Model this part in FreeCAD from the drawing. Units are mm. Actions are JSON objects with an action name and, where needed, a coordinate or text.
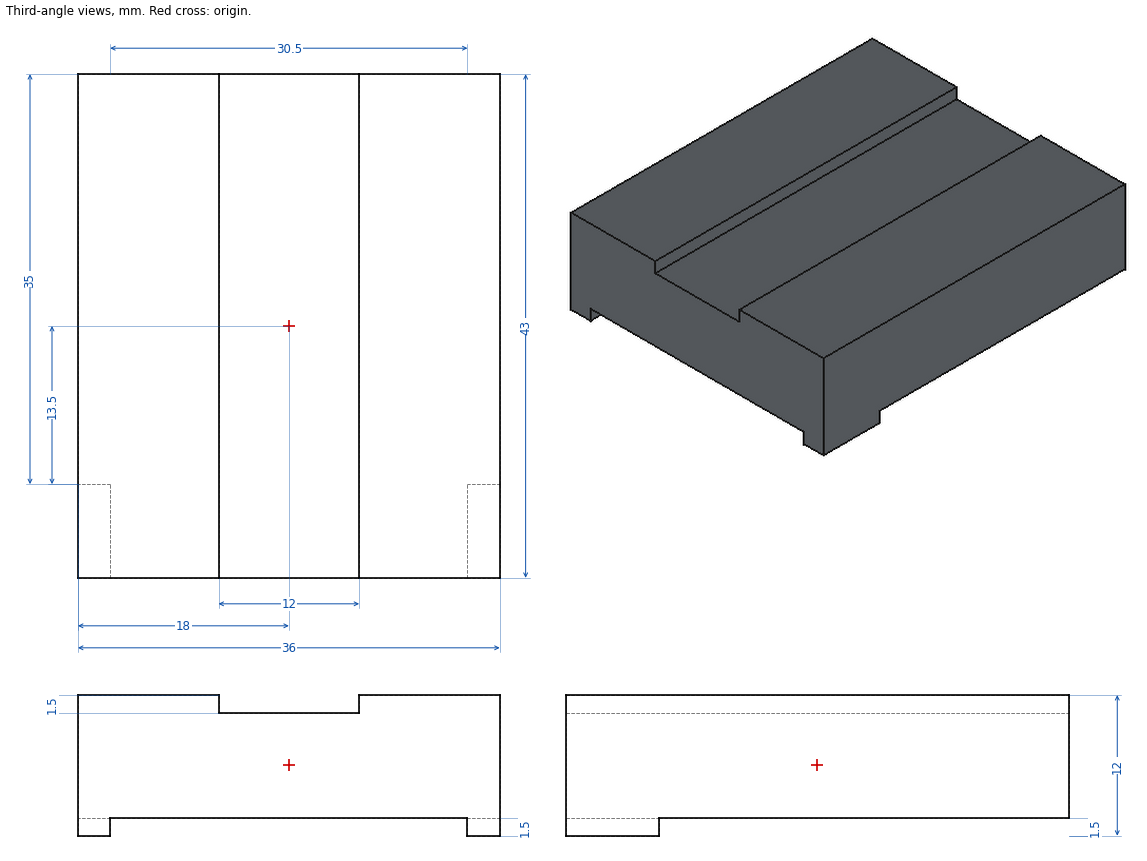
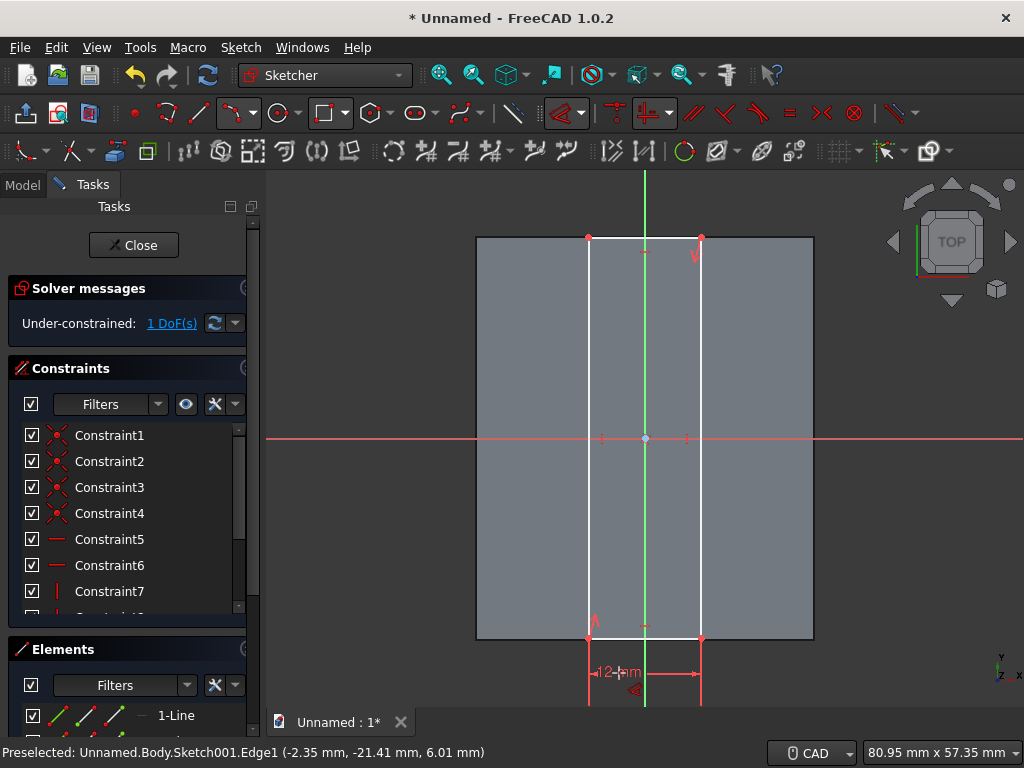
{"action": "left_click", "coordinate": [701, 519]}
{"action": "left_click", "coordinate": [735, 346]}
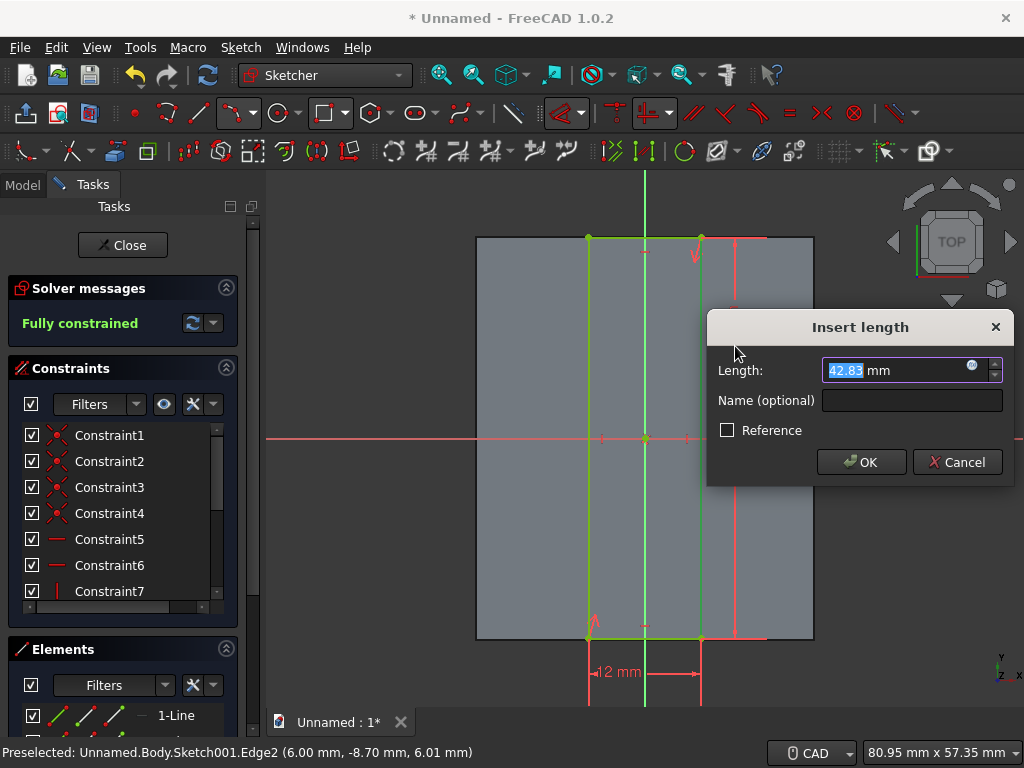
{"action": "type", "text": "43"}
{"action": "key", "text": "Return"}
{"action": "key", "text": "Escape"}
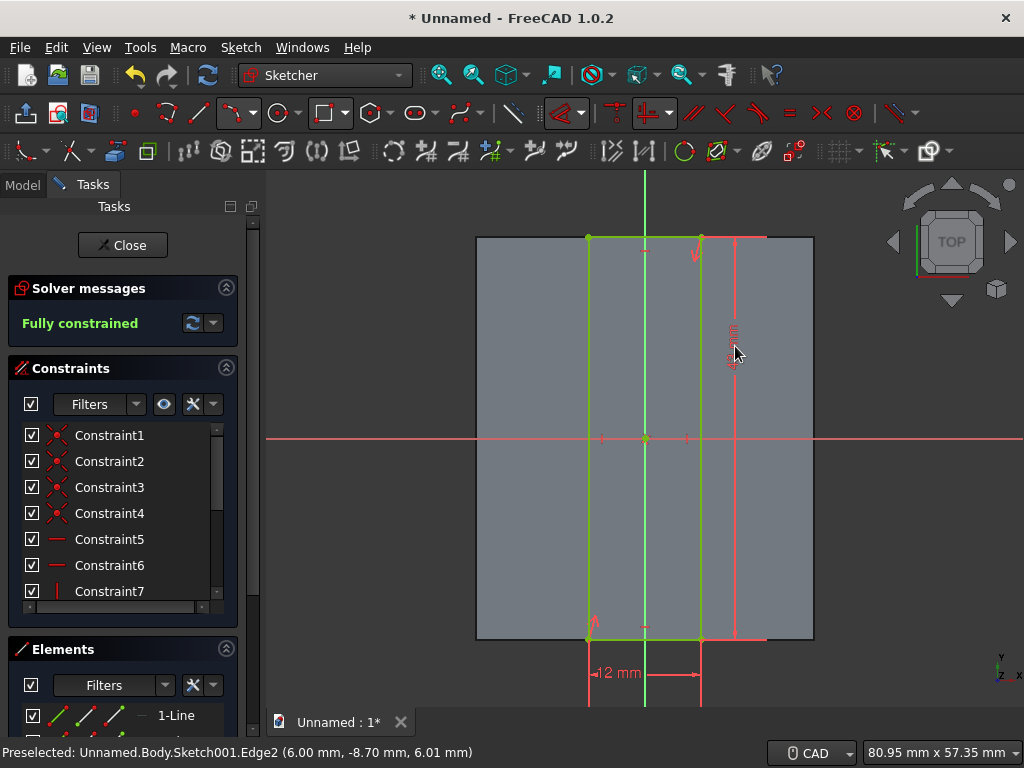
{"action": "left_click", "coordinate": [123, 245]}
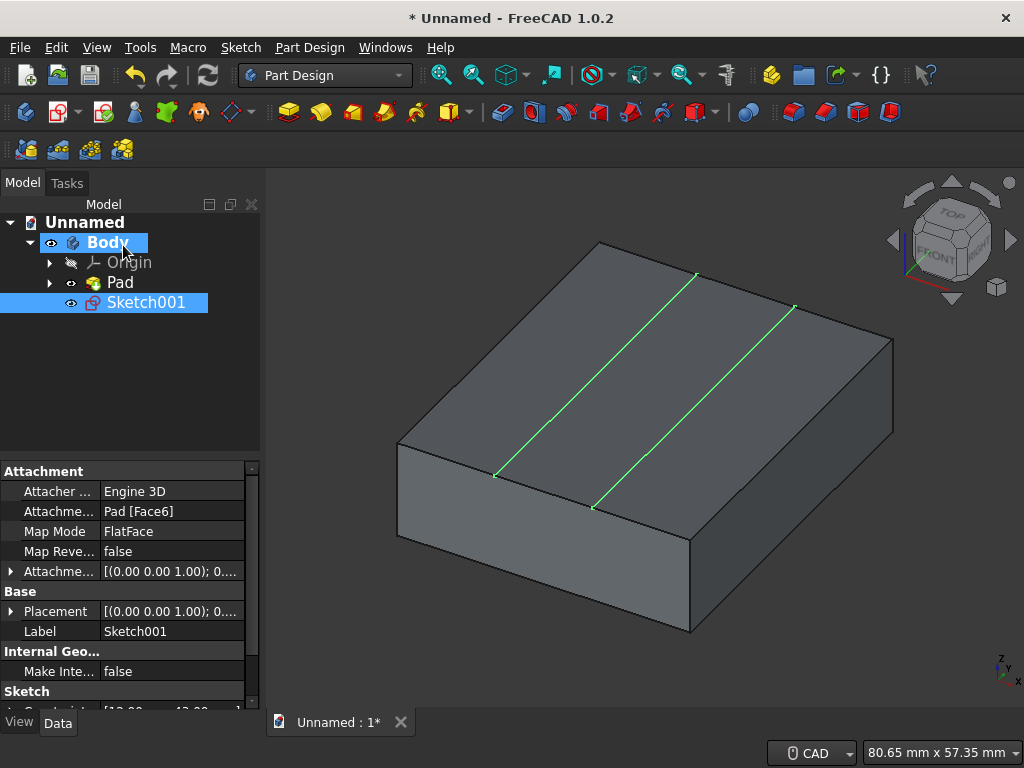
{"action": "left_click", "coordinate": [504, 112]}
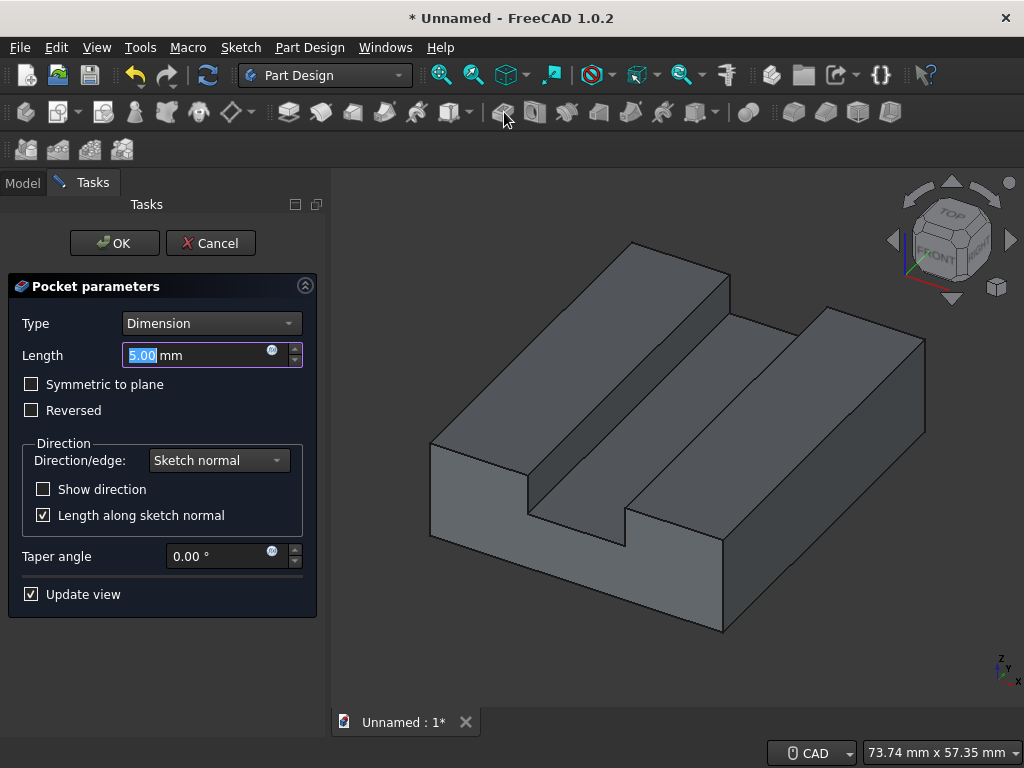
{"action": "type", "text": "1.5"}
{"action": "key", "text": "Tab"}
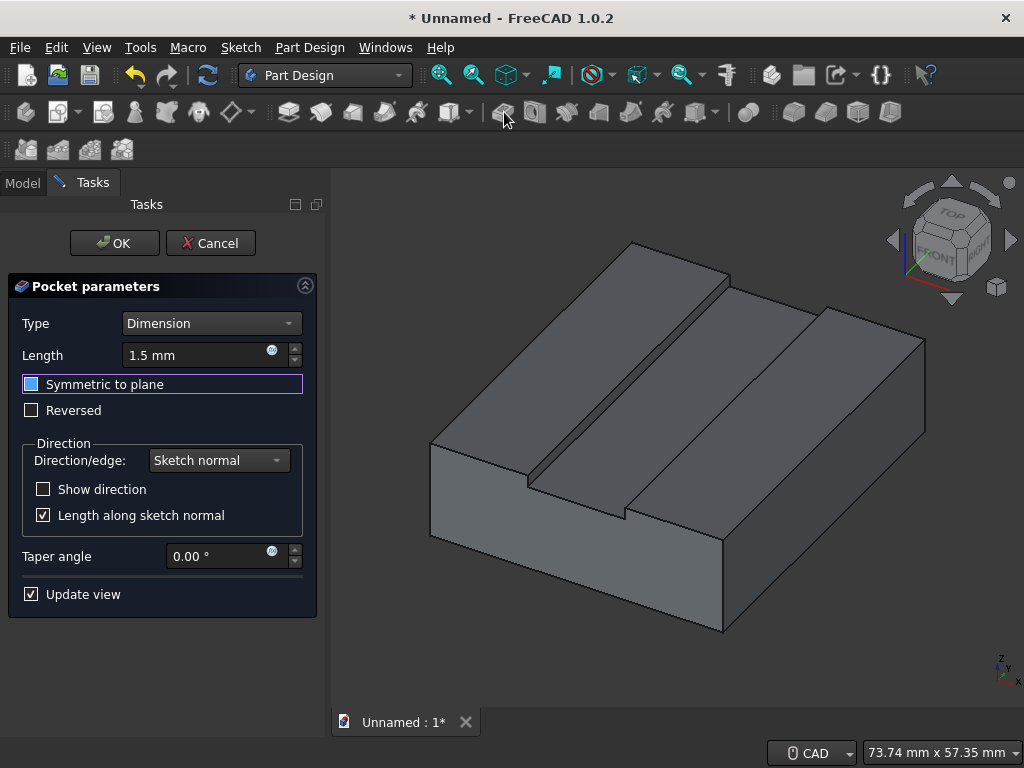
{"action": "left_click", "coordinate": [115, 243]}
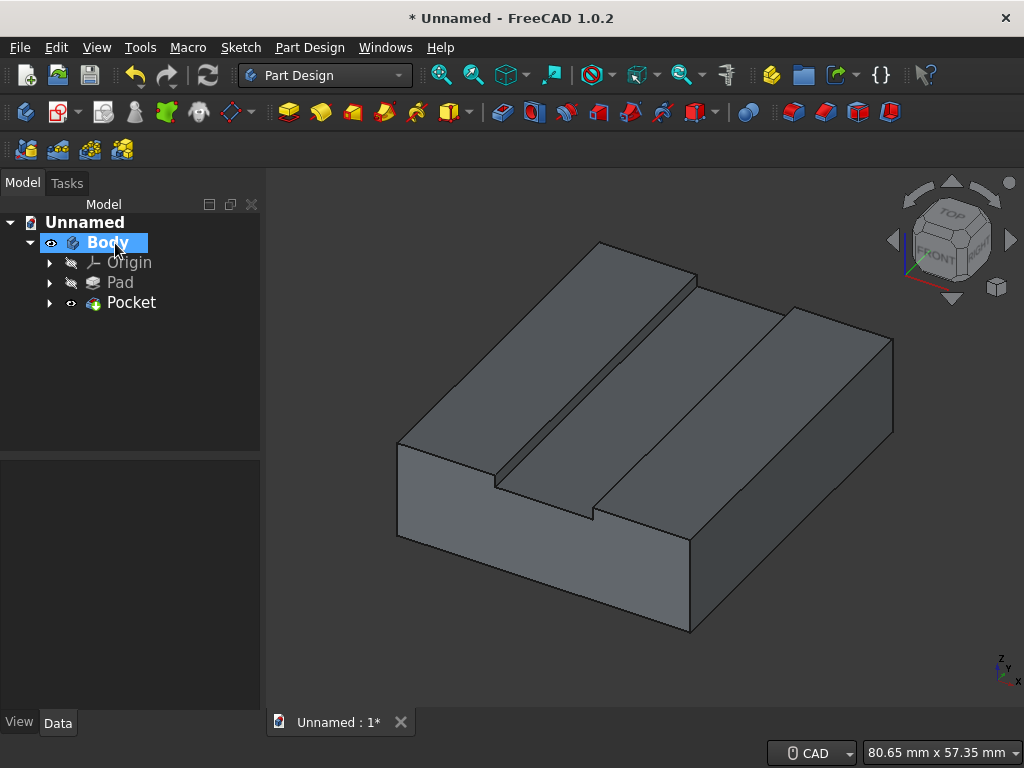
{"action": "key", "text": "5"}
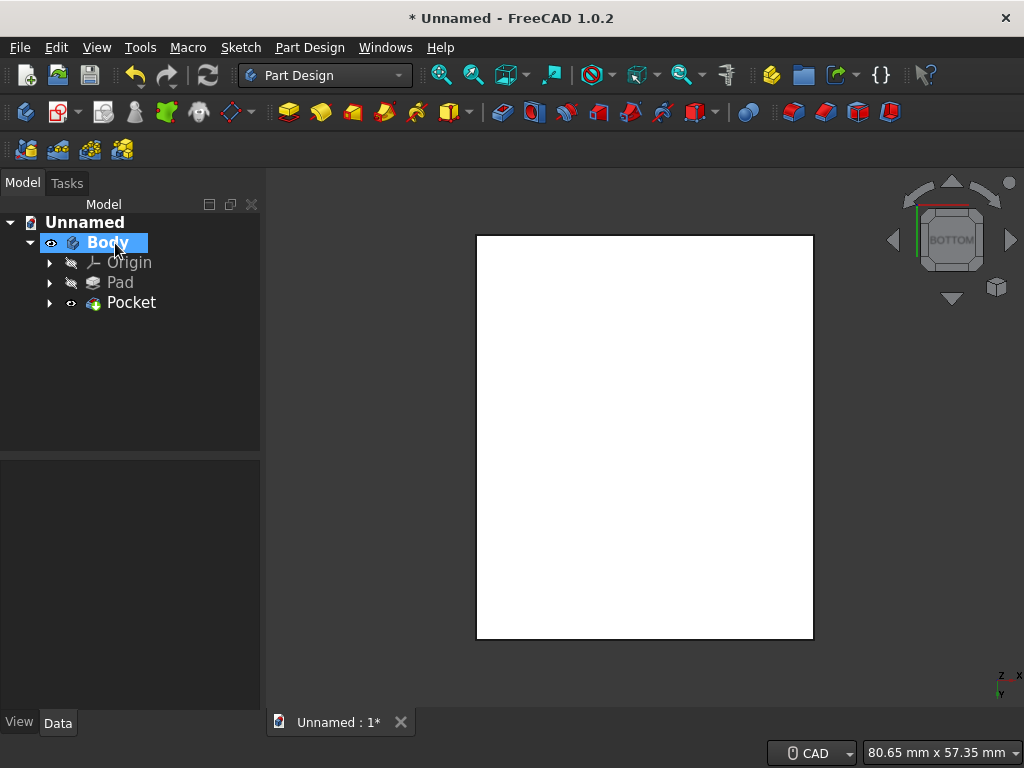
{"action": "left_click", "coordinate": [645, 436]}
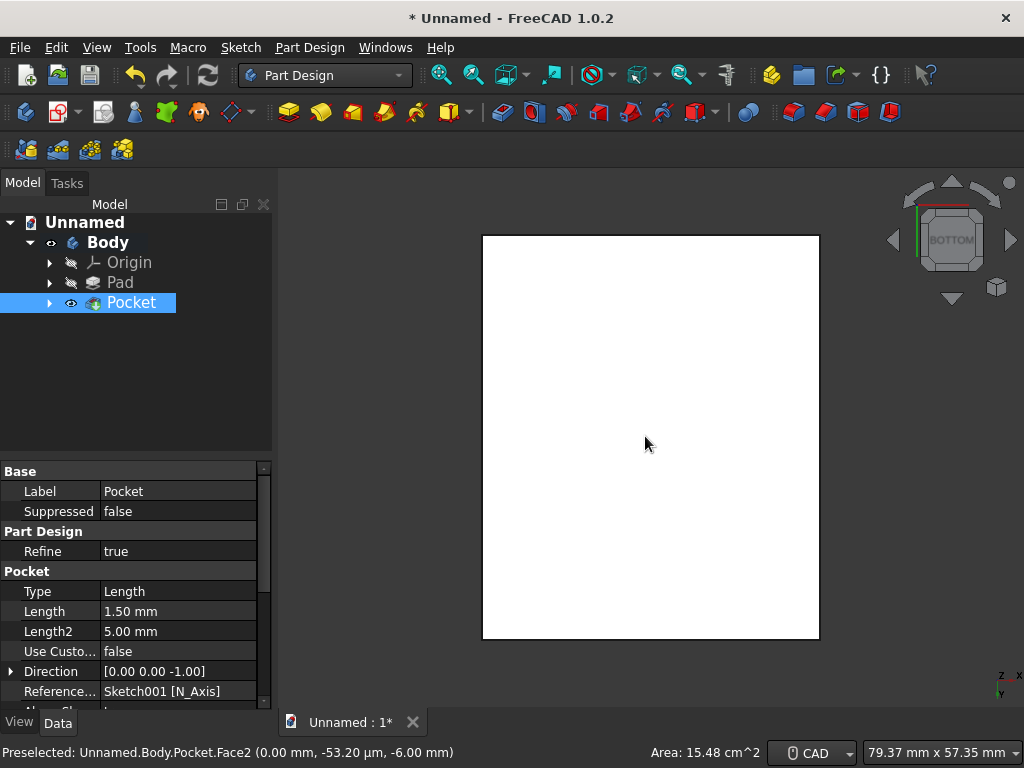
{"action": "left_click", "coordinate": [58, 112]}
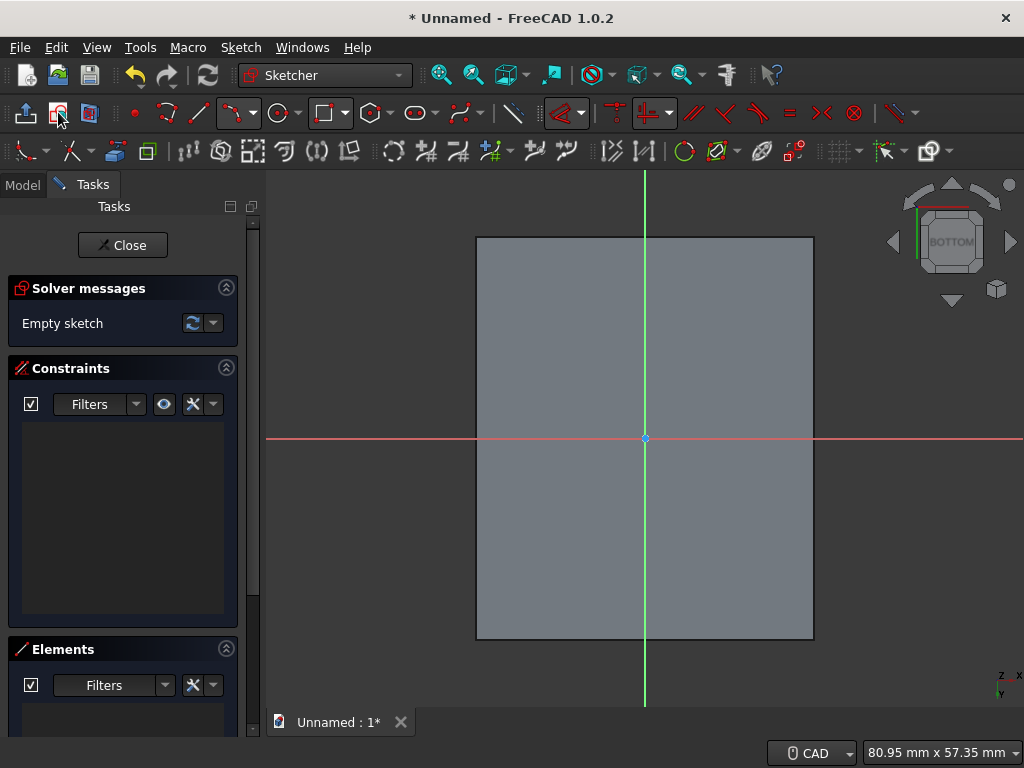
{"action": "key", "text": "g v"}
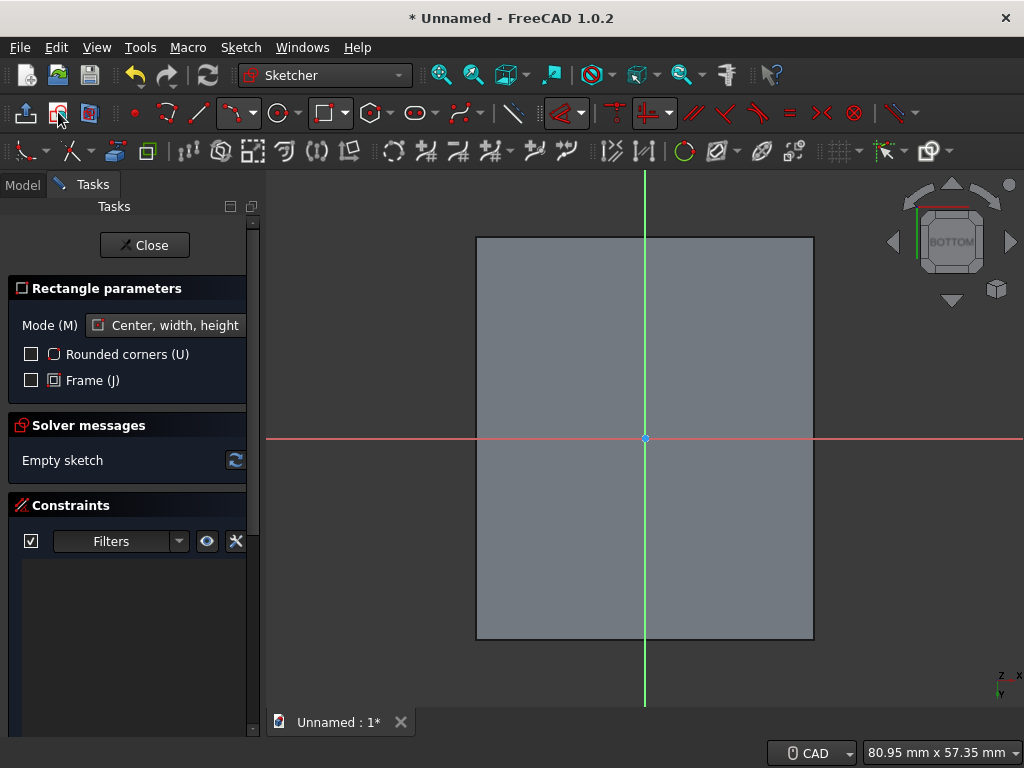
{"action": "left_click", "coordinate": [645, 438]}
{"action": "left_click", "coordinate": [788, 237]}
{"action": "key", "text": "Escape"}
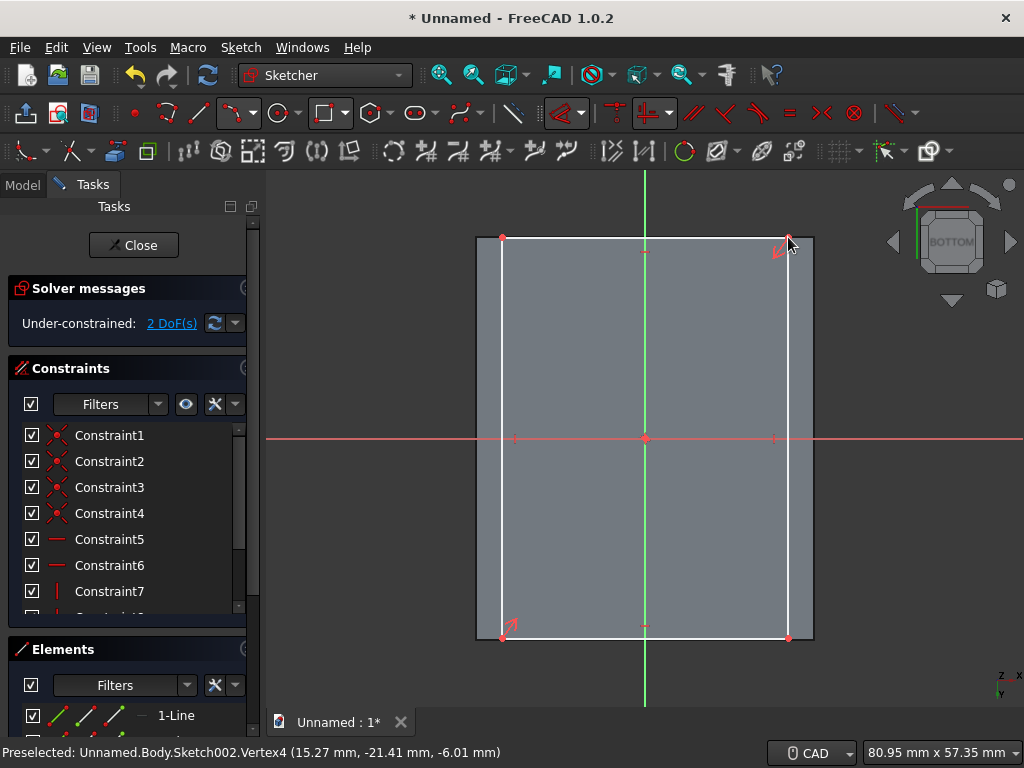
{"action": "key", "text": "d"}